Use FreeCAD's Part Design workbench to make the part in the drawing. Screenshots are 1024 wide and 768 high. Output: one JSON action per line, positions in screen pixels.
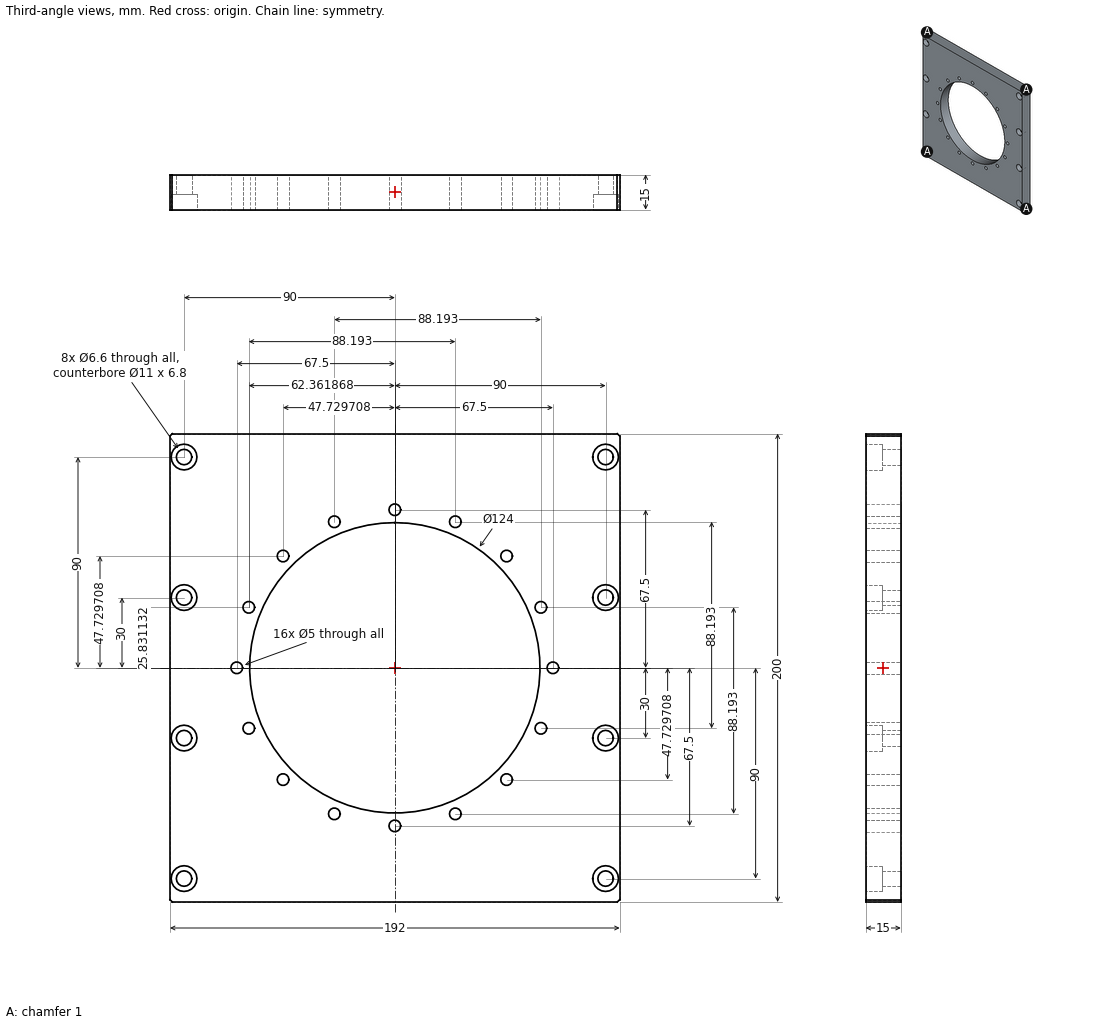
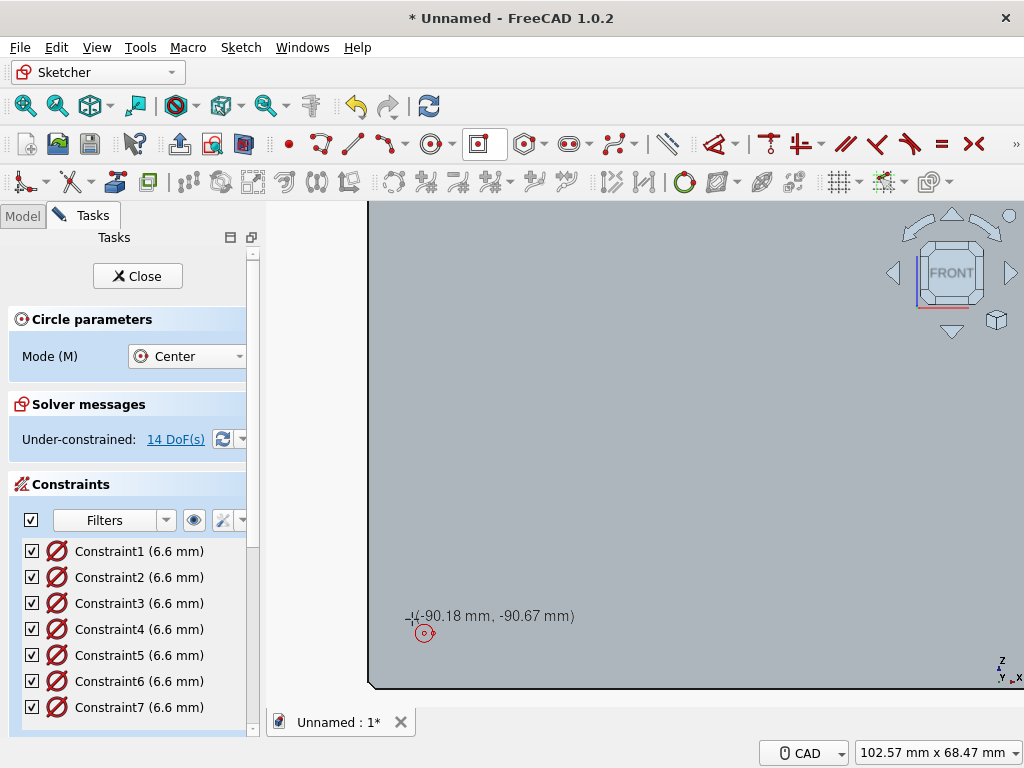
{"action": "scroll", "coordinate": [412, 619], "scroll_direction": "down", "scroll_amount": 7}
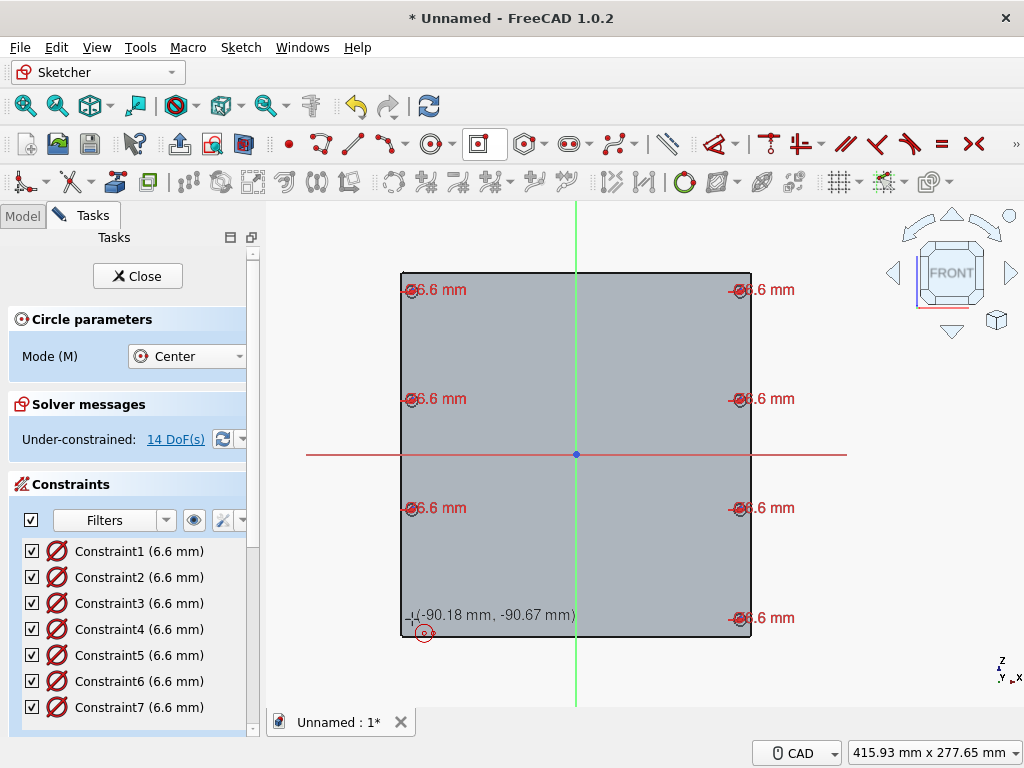
{"action": "left_click", "coordinate": [412, 619]}
{"action": "mouse_move", "coordinate": [417, 615]}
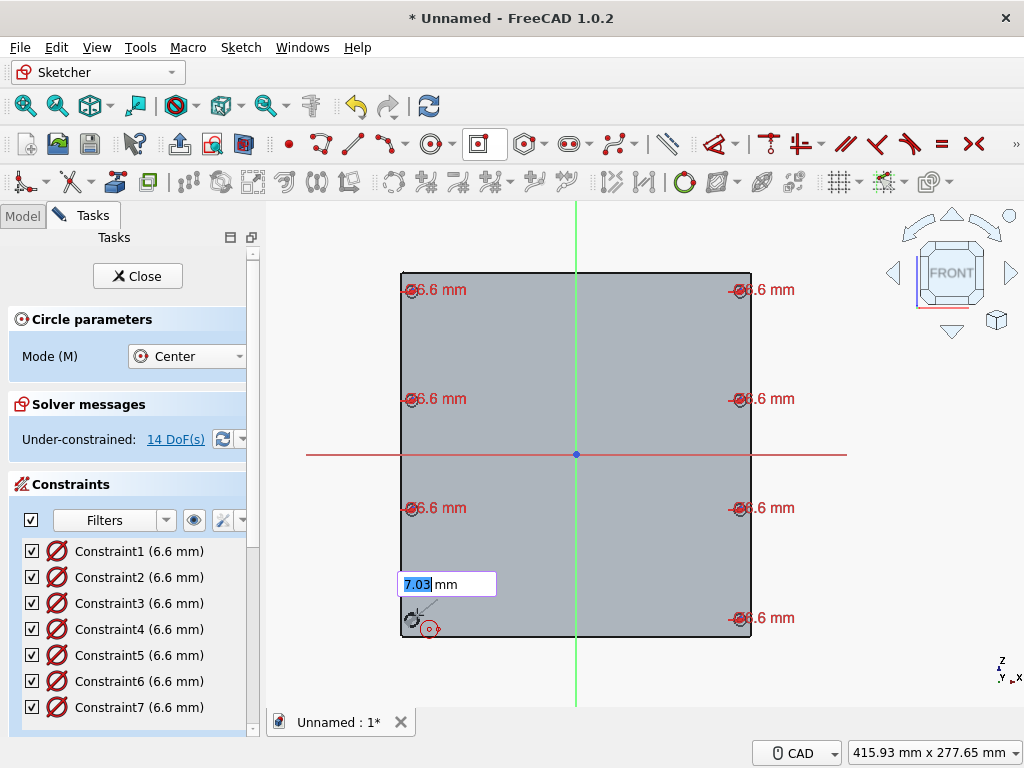
{"action": "type", "text": "6.6"}
{"action": "key", "text": "Return"}
{"action": "key", "text": "Escape"}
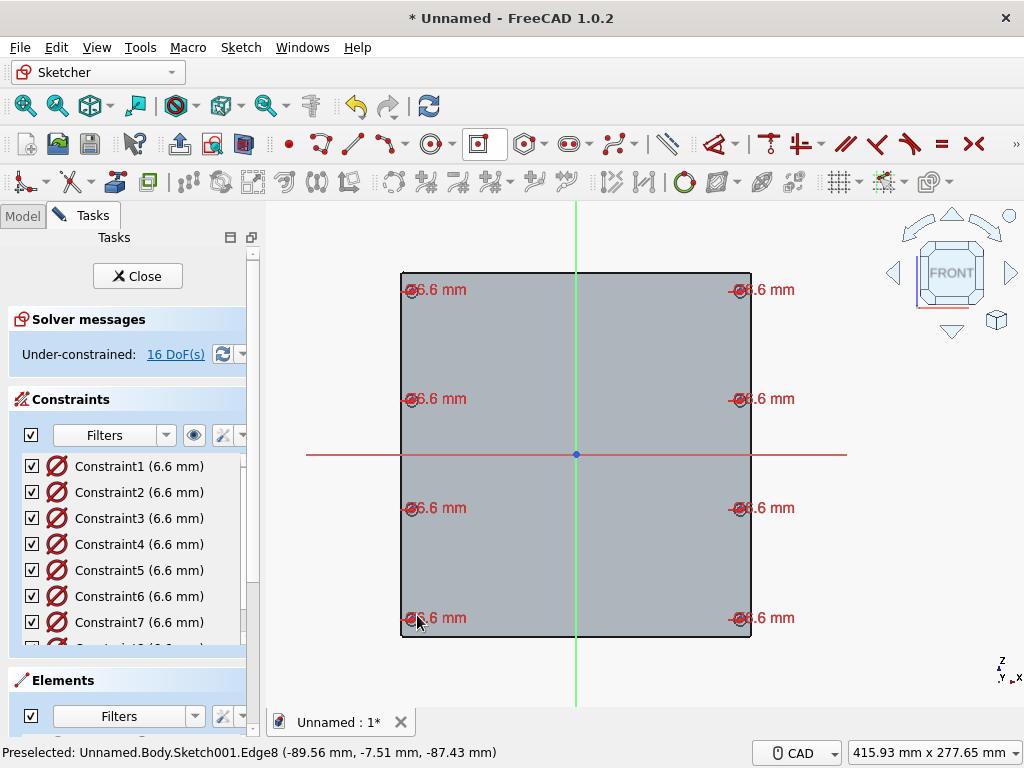
{"action": "left_click", "coordinate": [412, 292]}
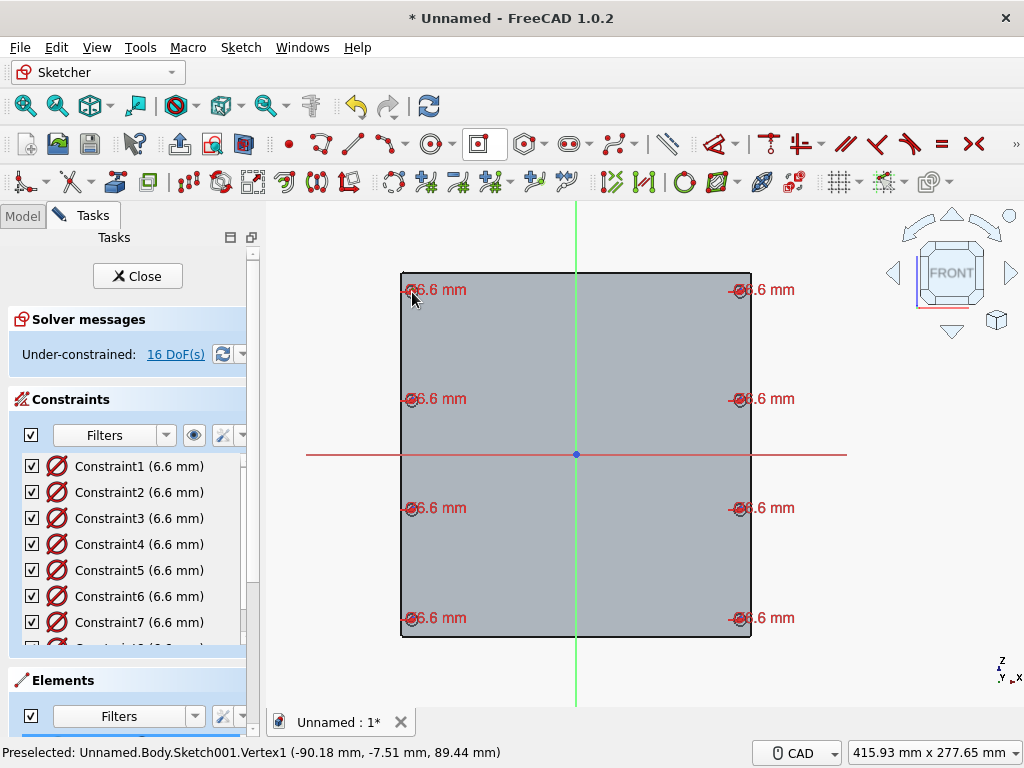
{"action": "left_click", "coordinate": [412, 401]}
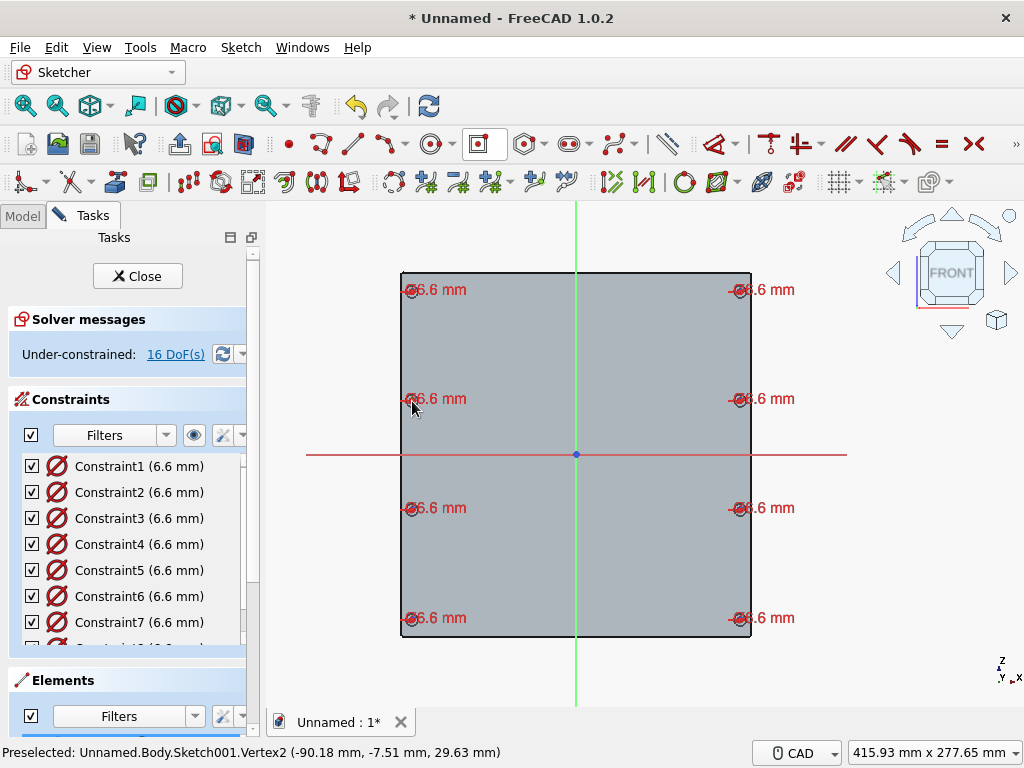
{"action": "left_click", "coordinate": [824, 144]}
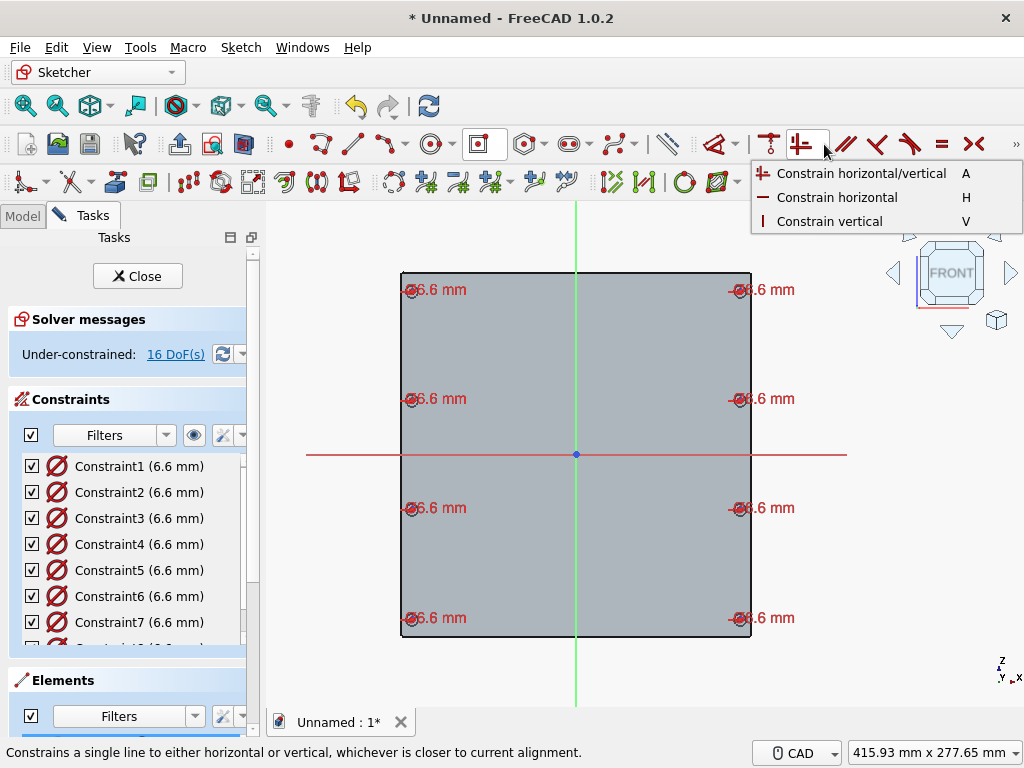
{"action": "left_click", "coordinate": [887, 221]}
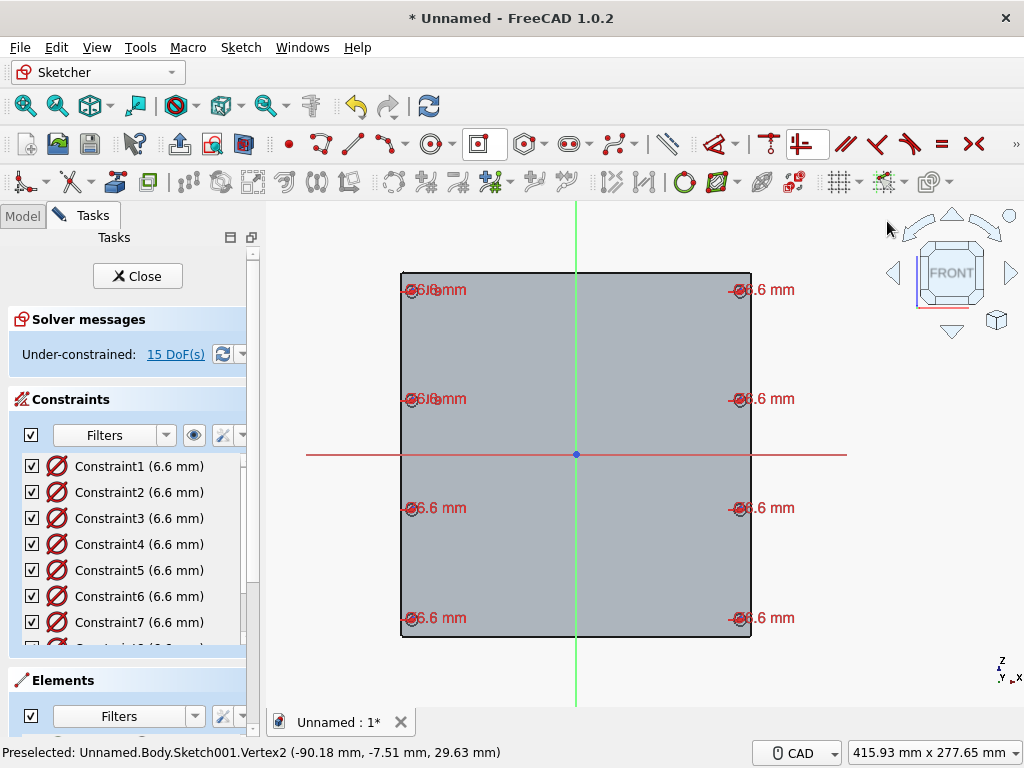
{"action": "left_click", "coordinate": [412, 401]}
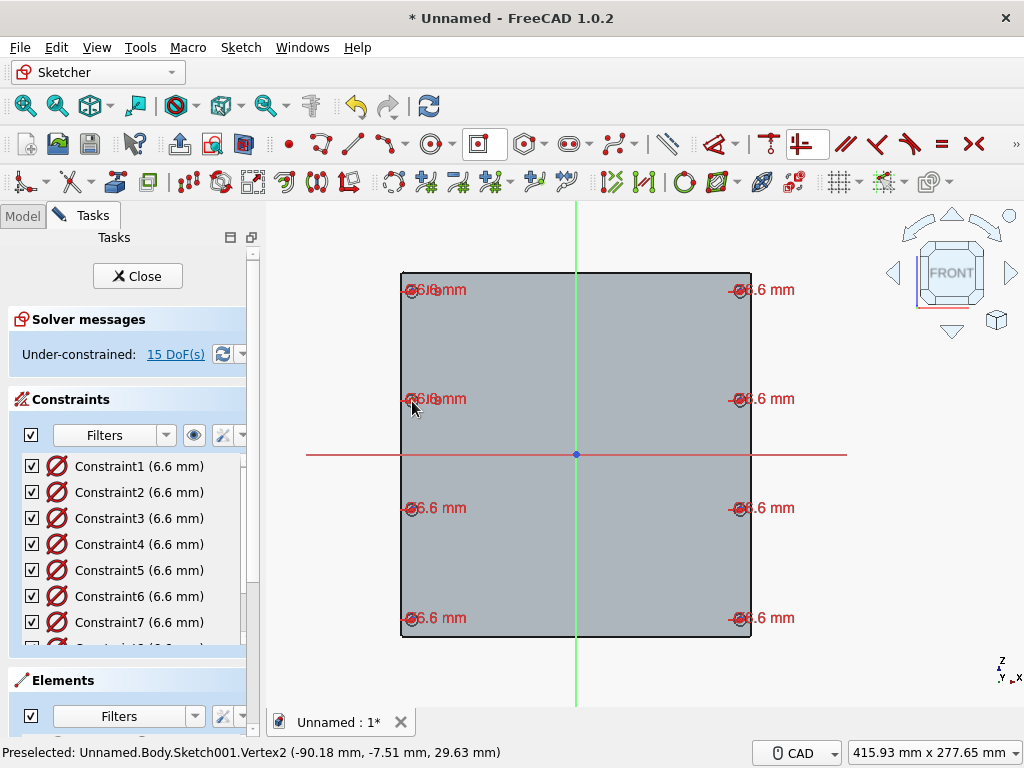
{"action": "left_click", "coordinate": [740, 401]}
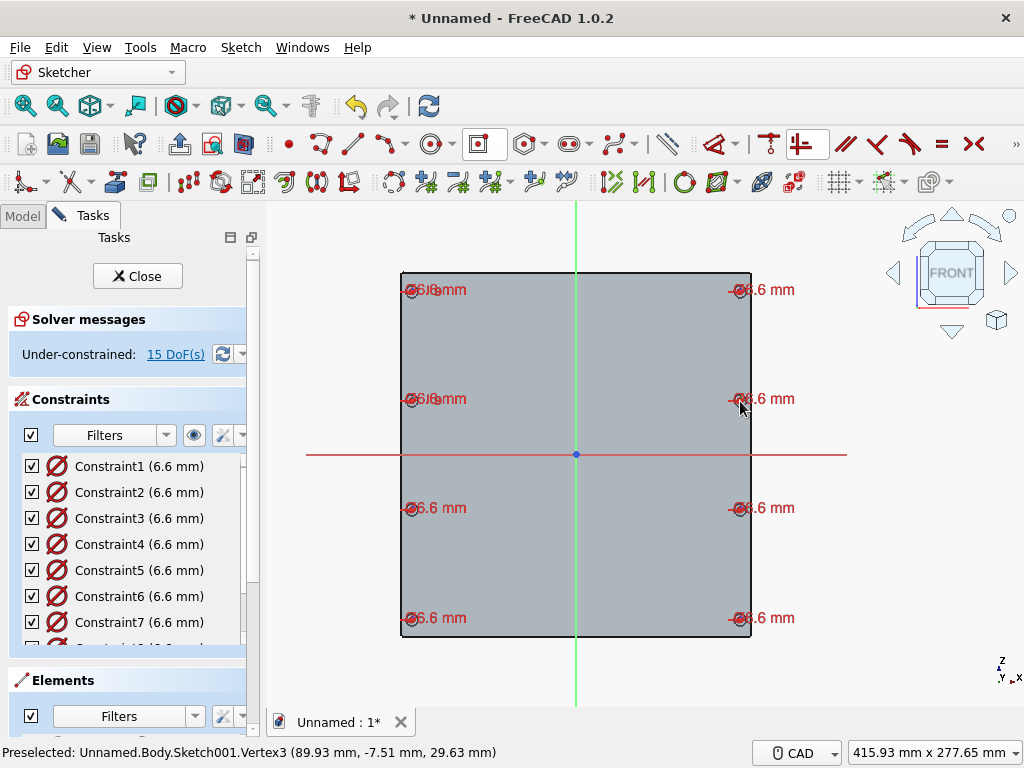
{"action": "key", "text": "h"}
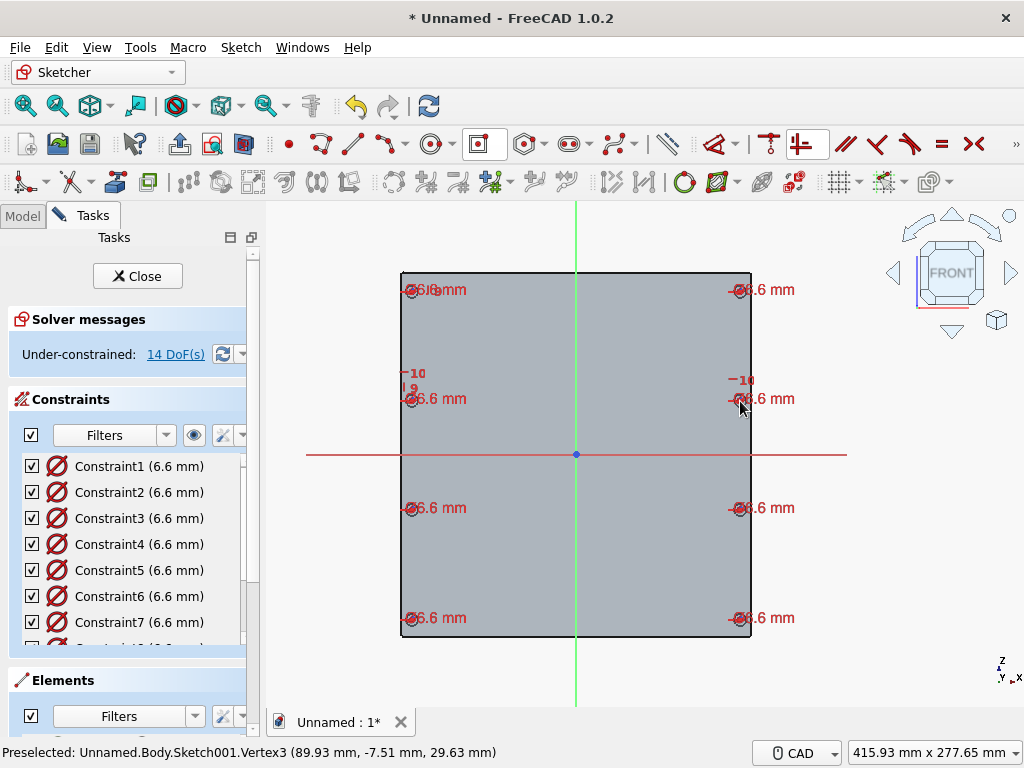
{"action": "left_click", "coordinate": [740, 401]}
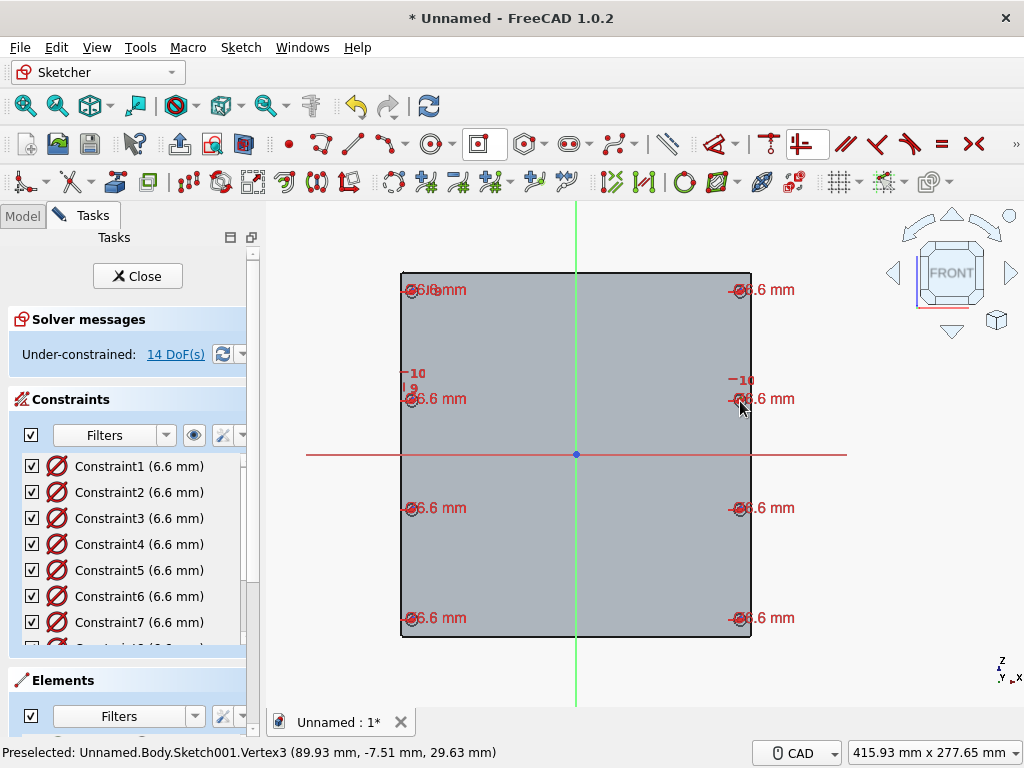
{"action": "left_click", "coordinate": [740, 292]}